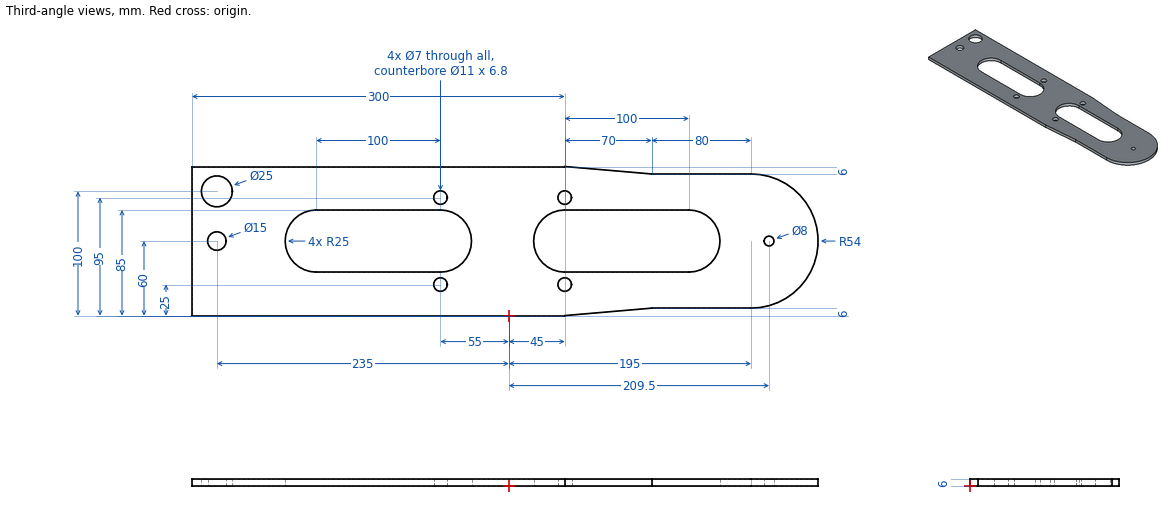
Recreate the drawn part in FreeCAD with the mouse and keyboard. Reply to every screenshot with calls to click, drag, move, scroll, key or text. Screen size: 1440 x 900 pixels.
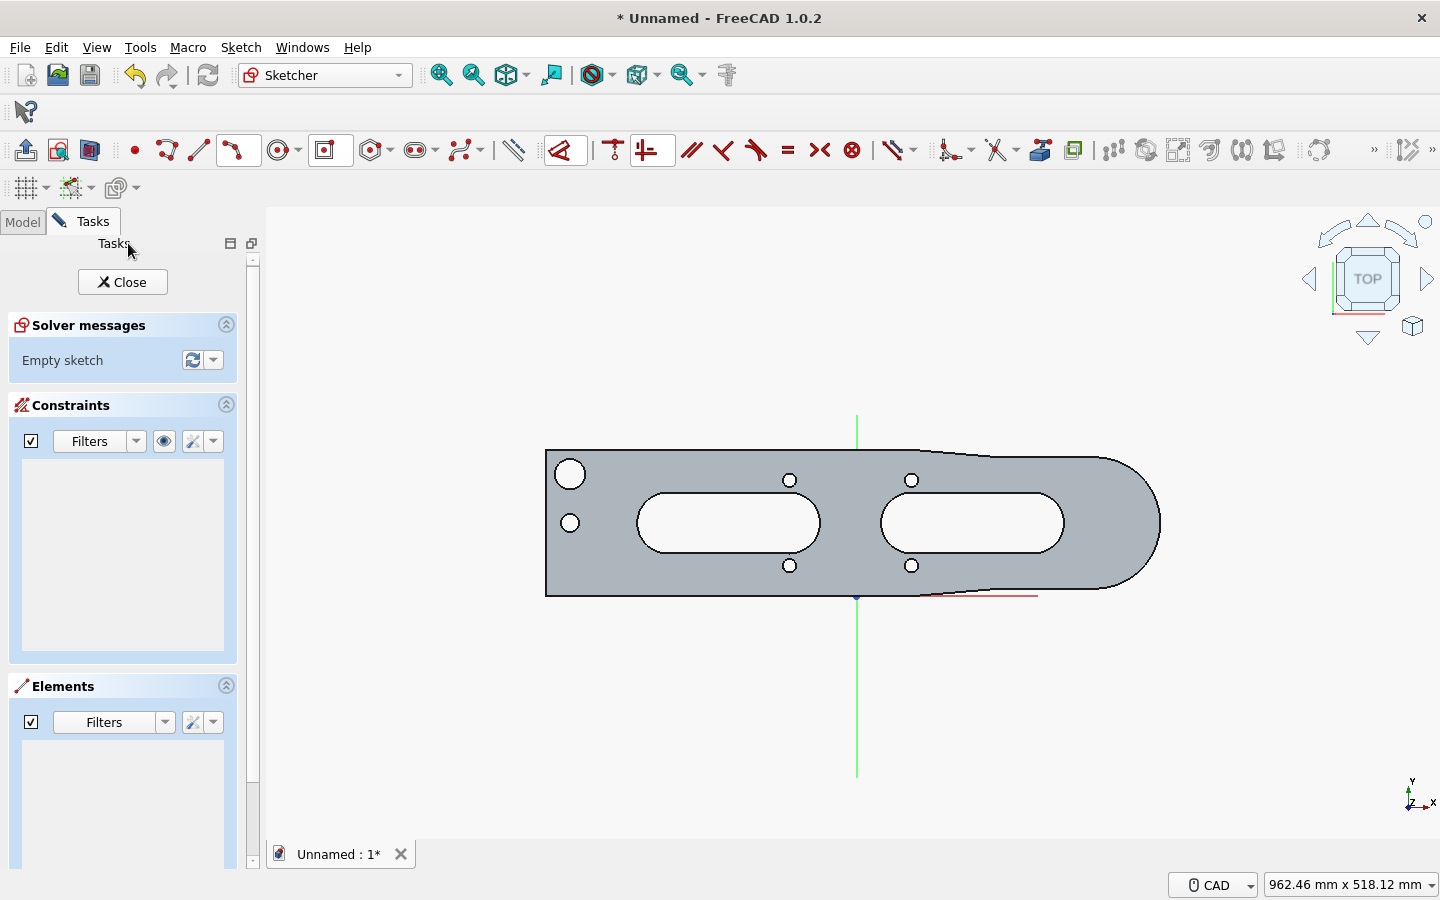
click(90, 150)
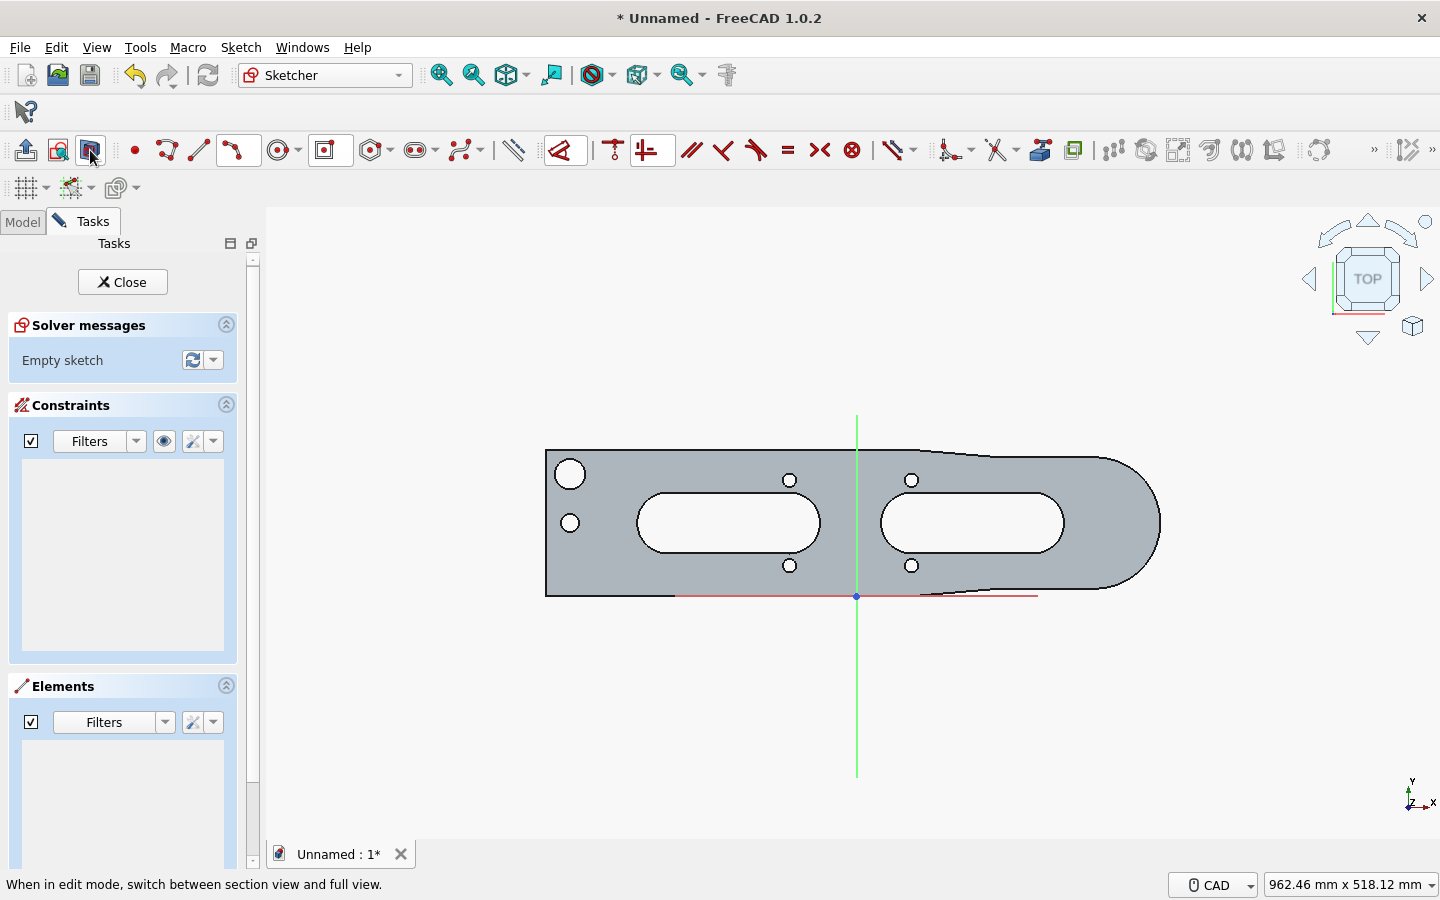
scroll(1129, 523, up, 15)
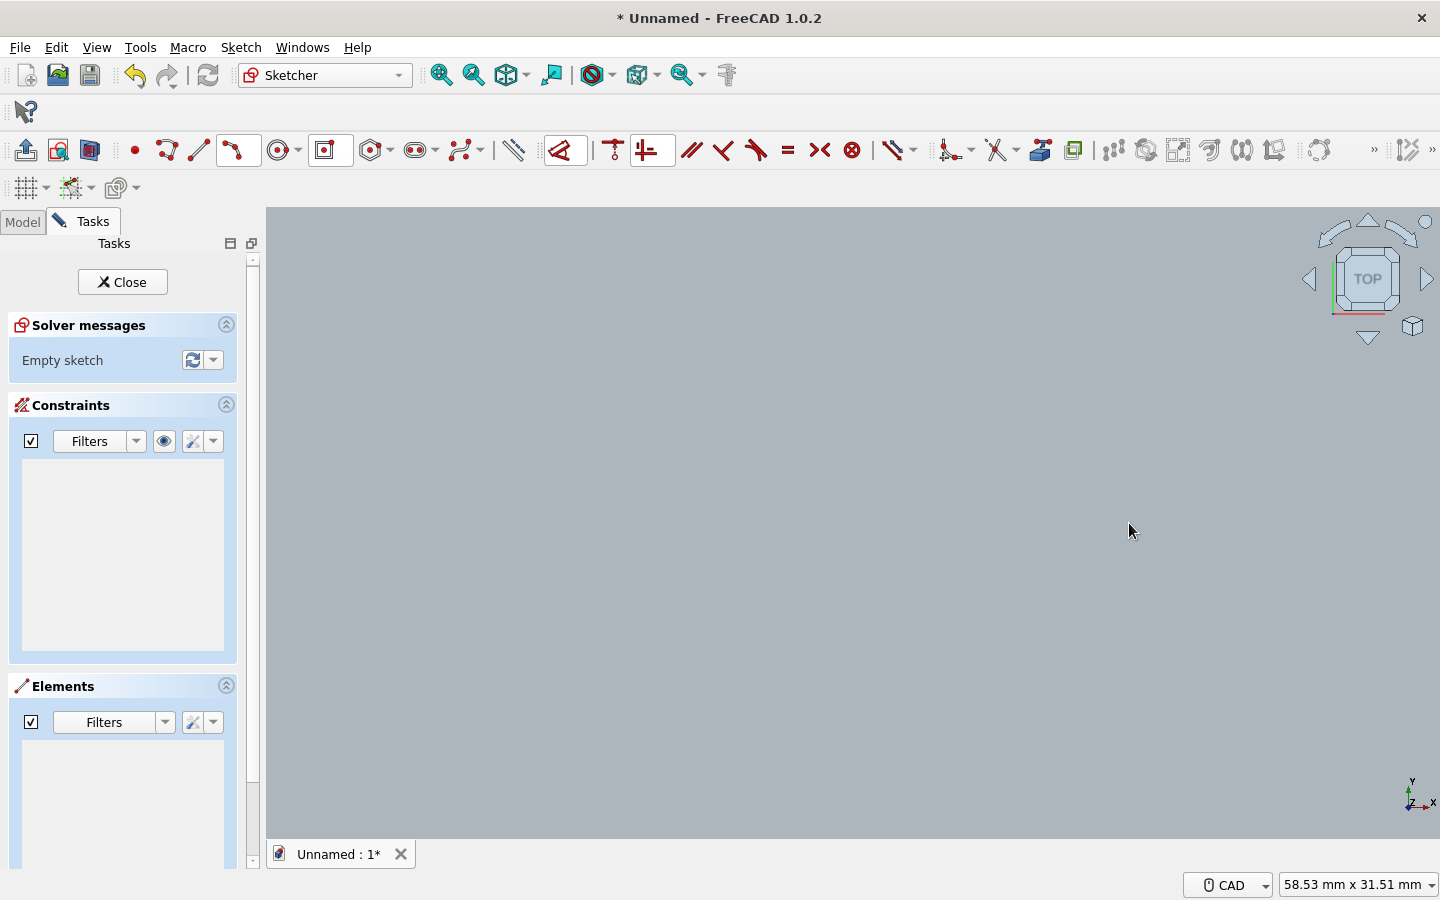
scroll(772, 506, up, 4)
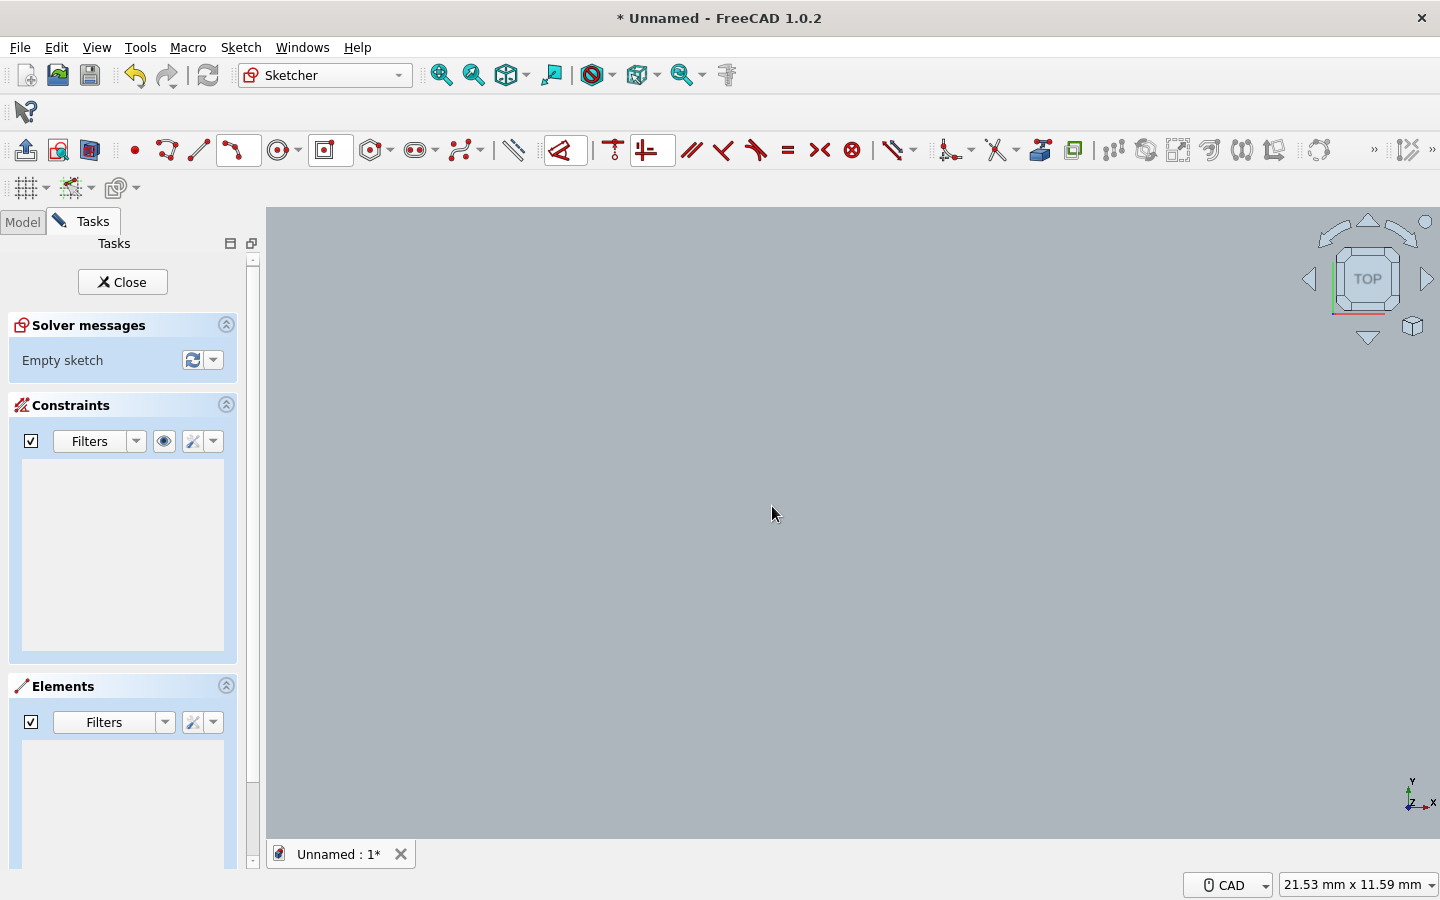
key(g)
key(c)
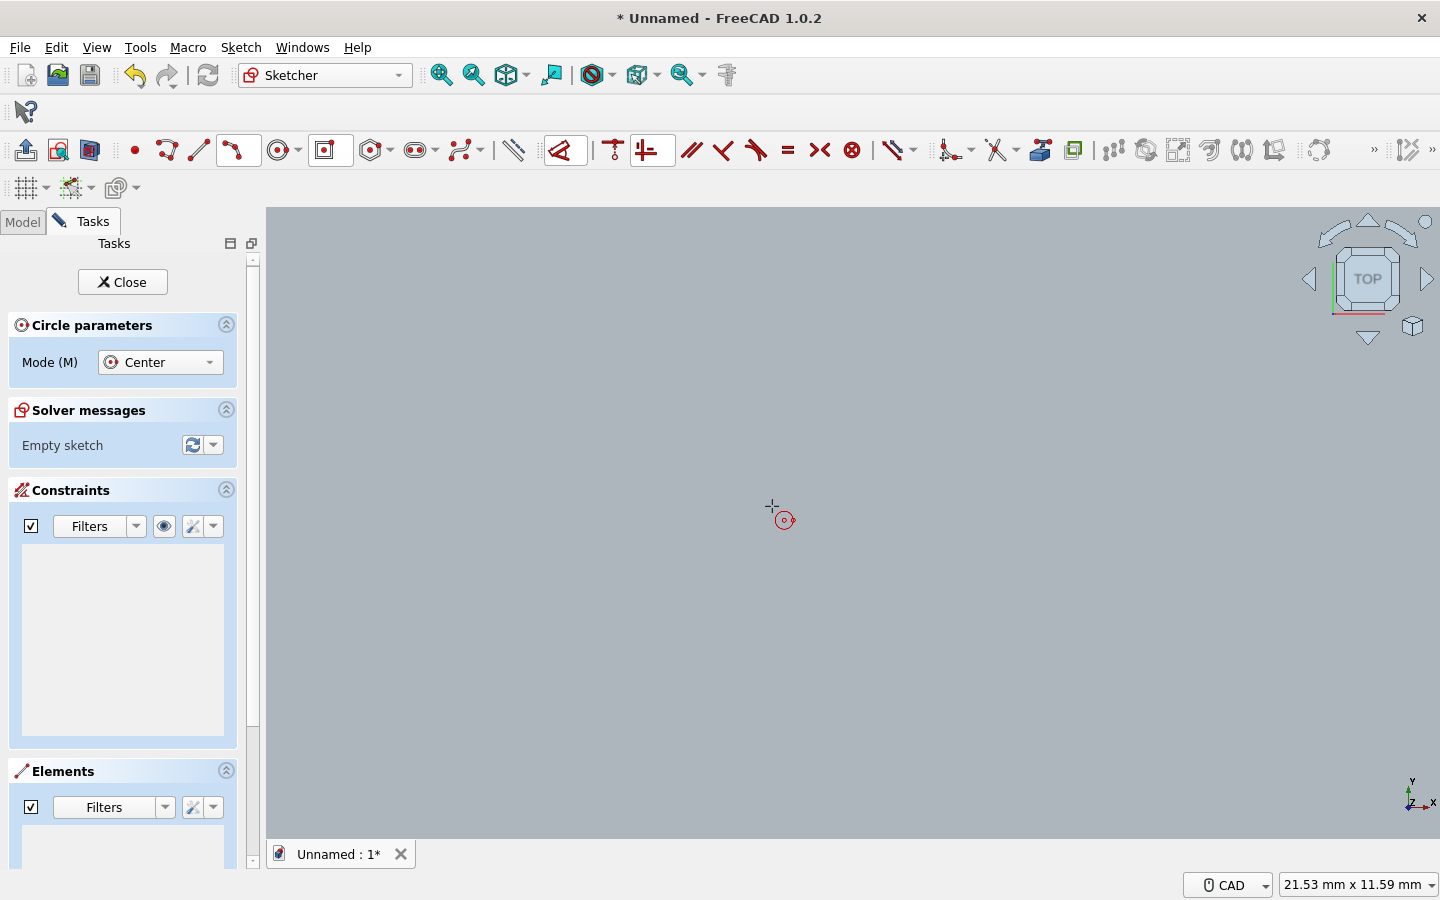
click(784, 522)
move(938, 368)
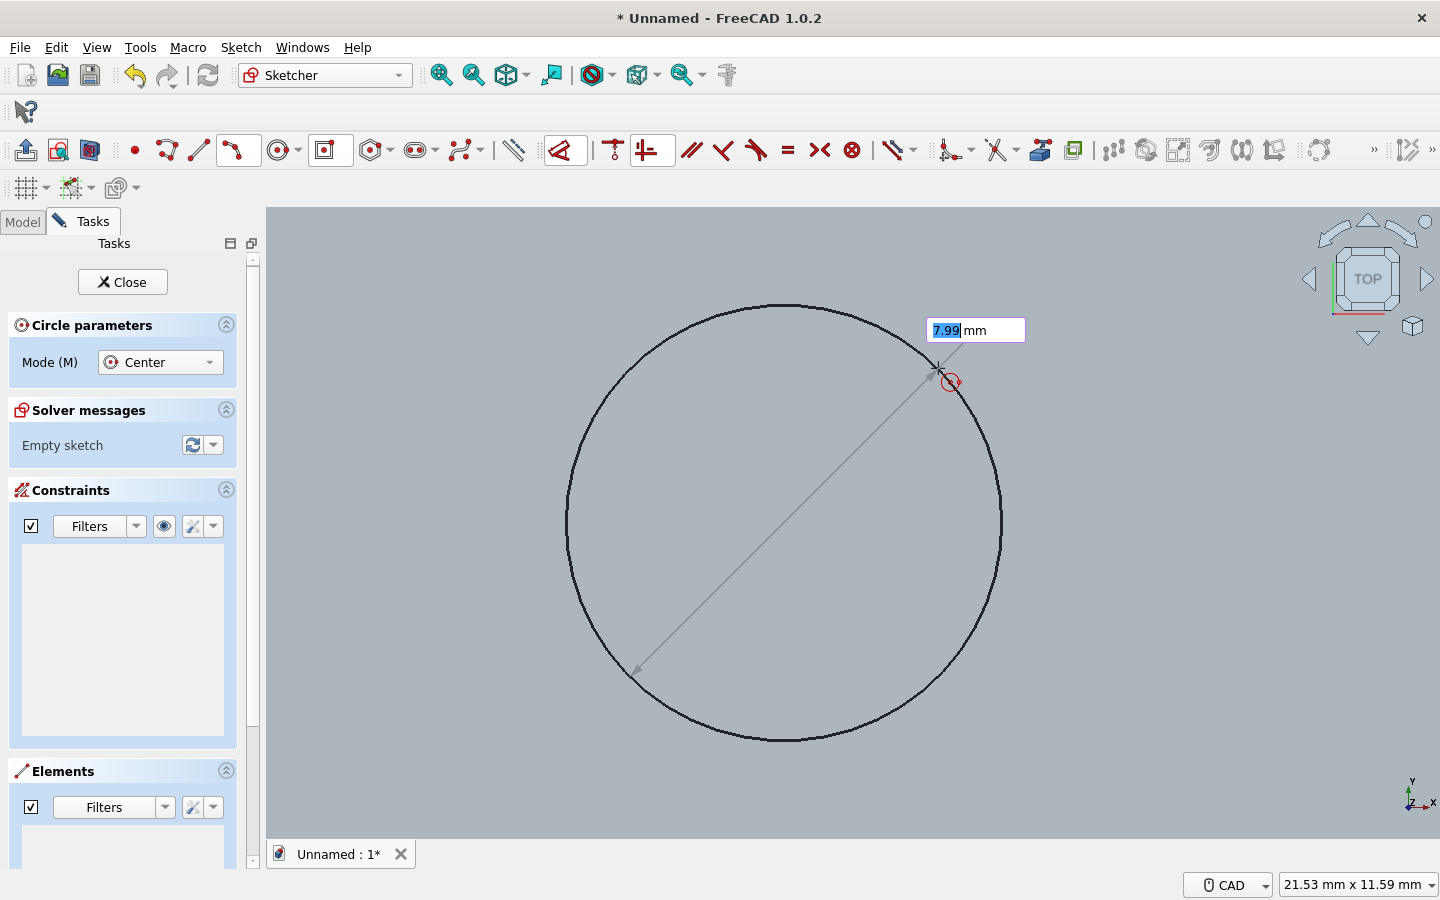
text(8)
key(Return)
key(Escape)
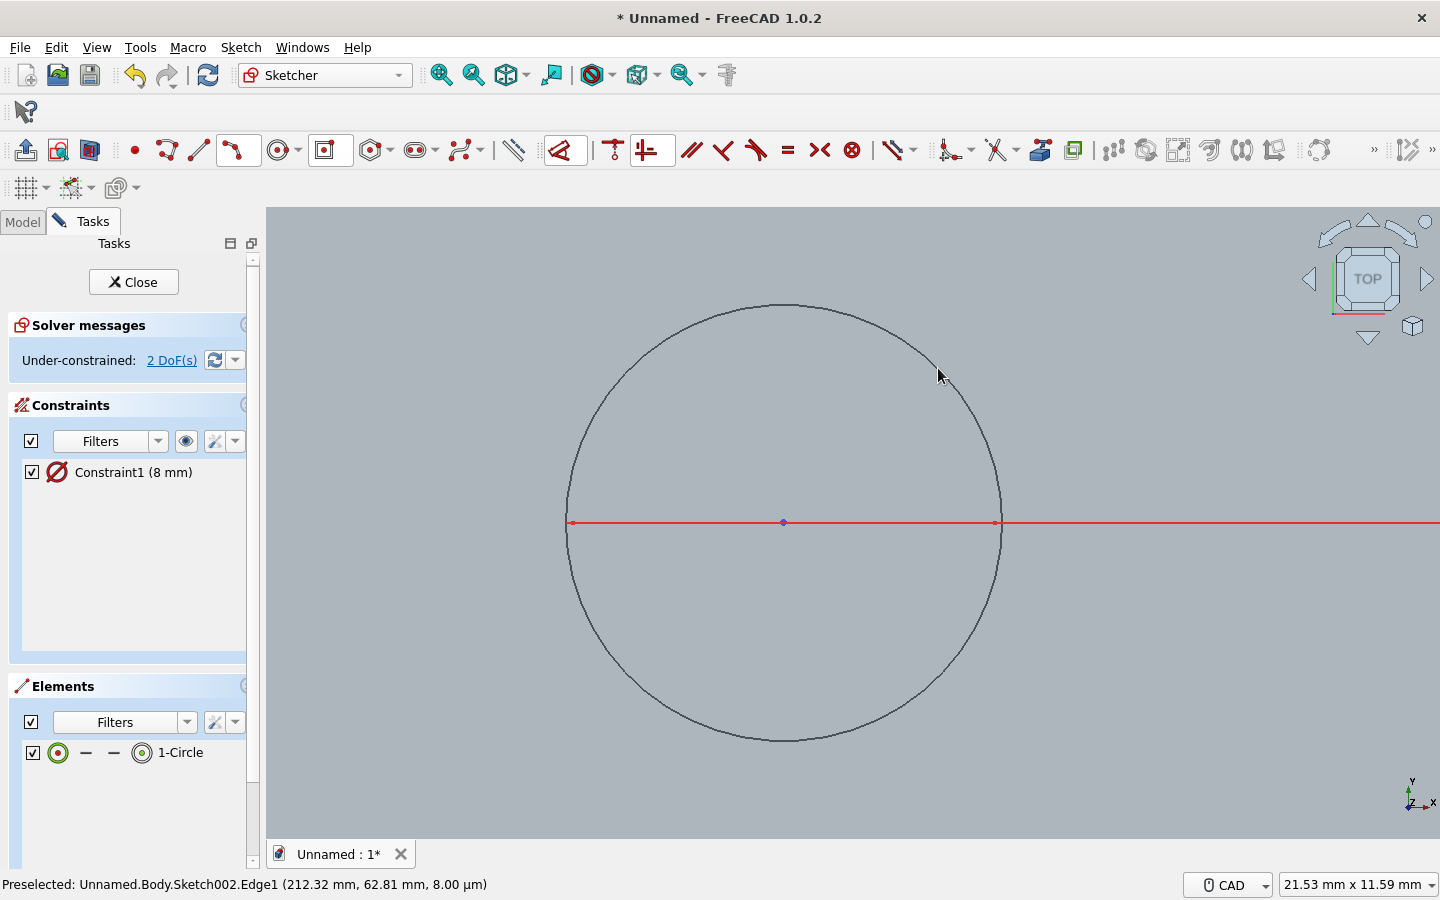
click(784, 523)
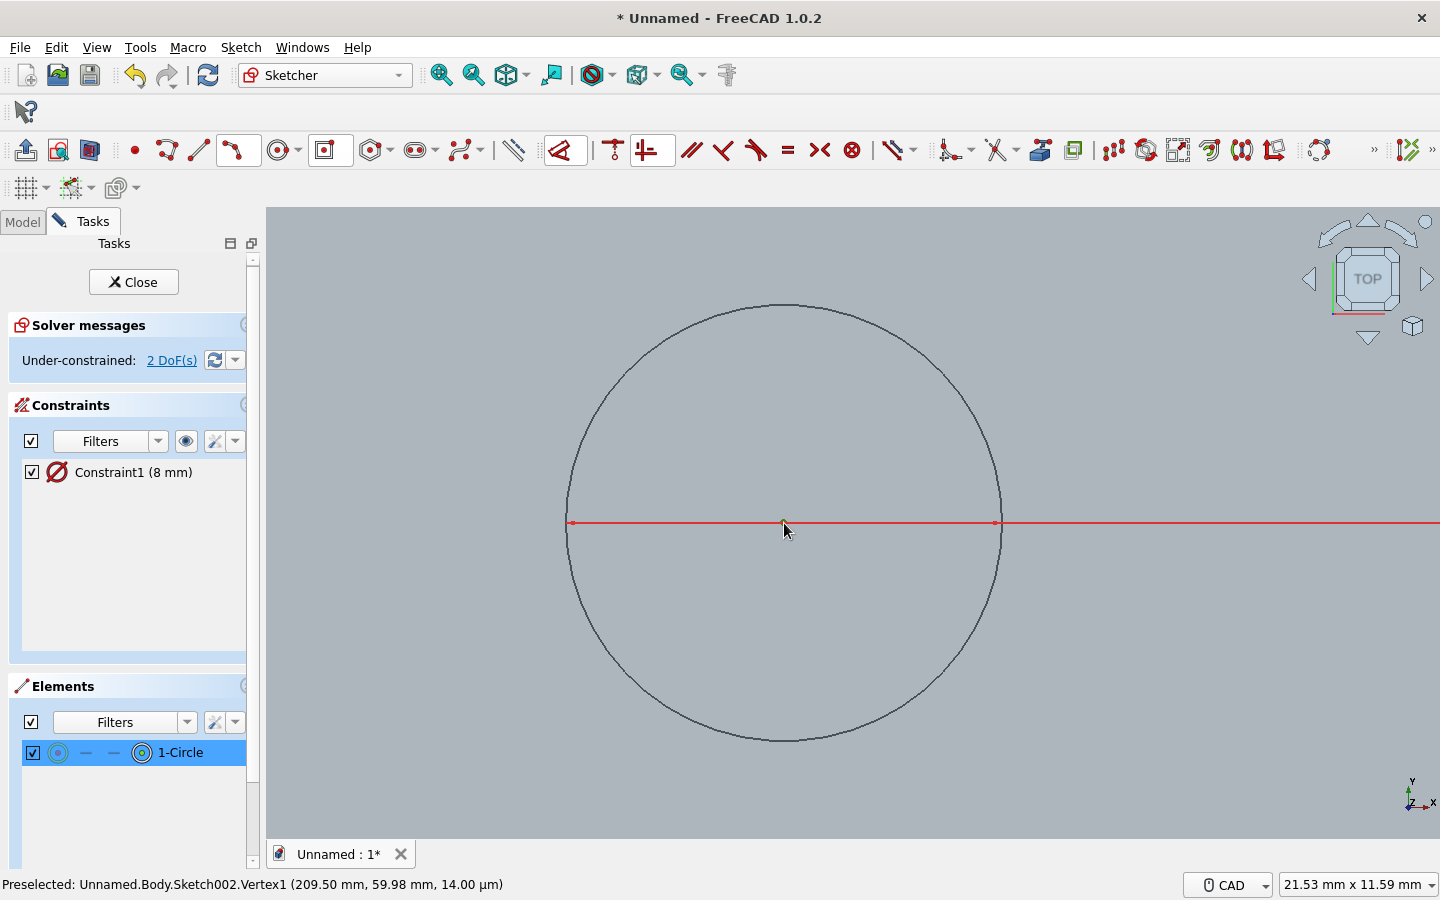
key(i)